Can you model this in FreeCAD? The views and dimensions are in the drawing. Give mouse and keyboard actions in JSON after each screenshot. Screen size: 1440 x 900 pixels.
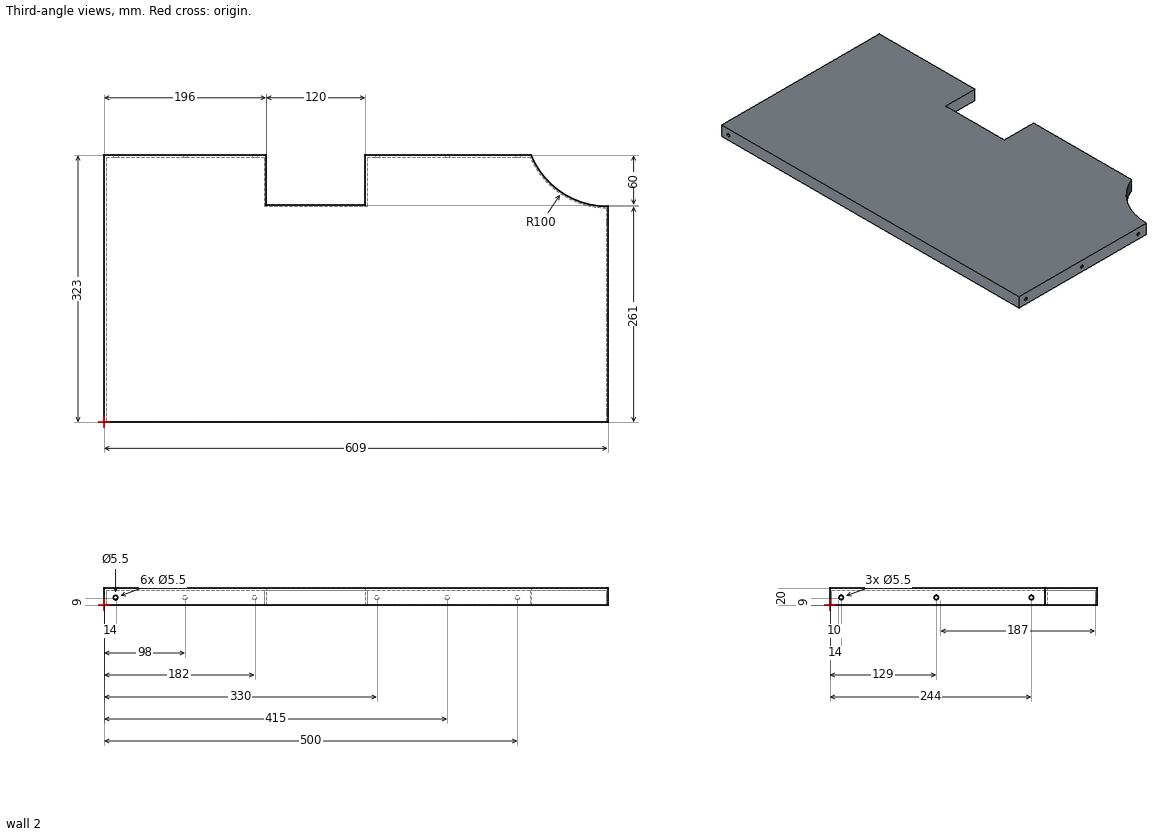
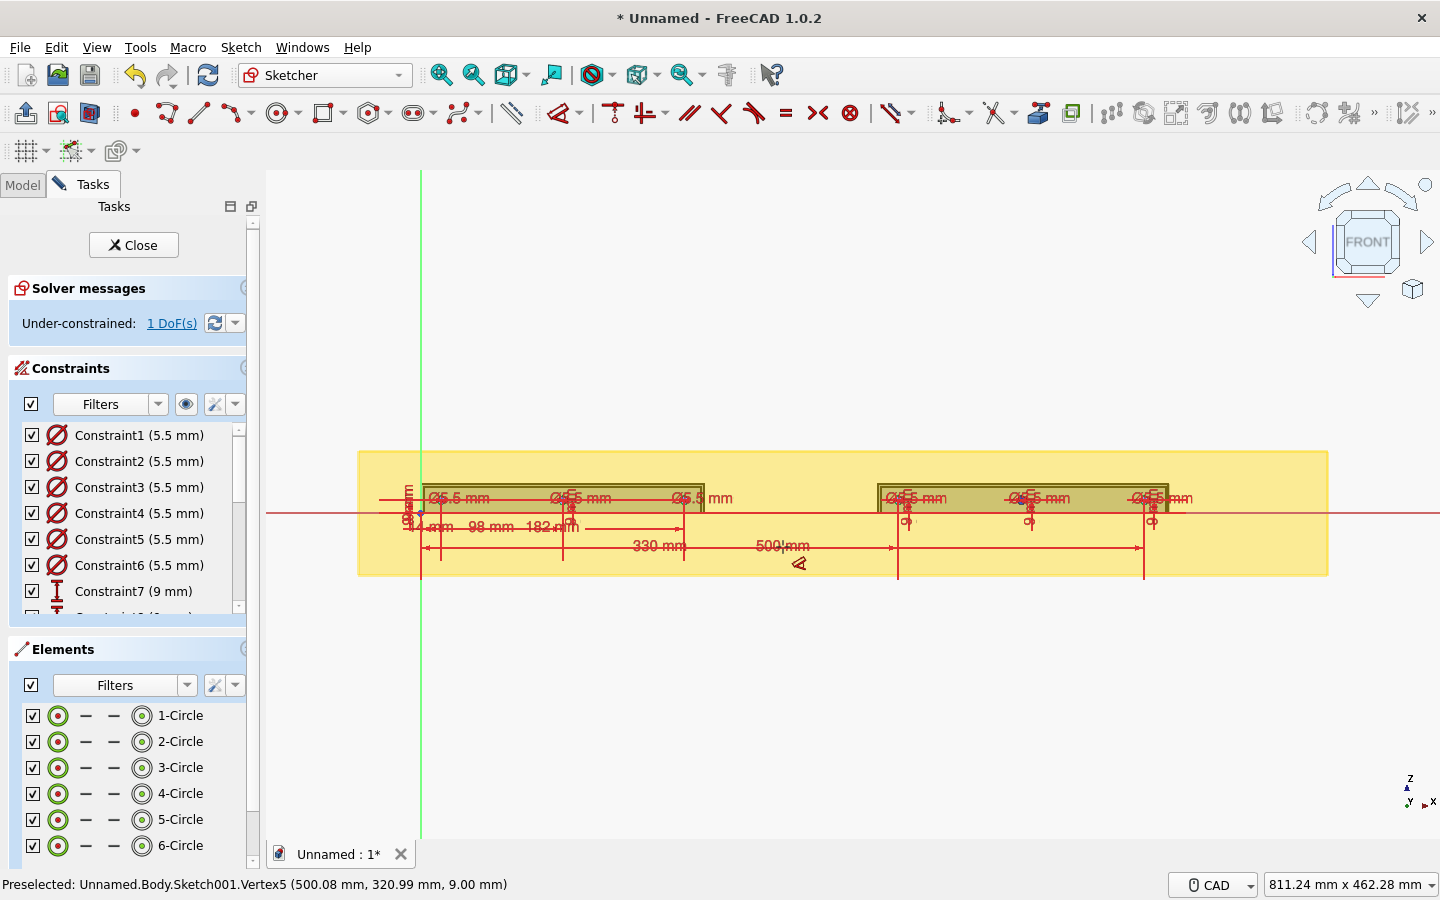
{"action": "left_click", "coordinate": [1021, 500]}
{"action": "left_click", "coordinate": [859, 547]}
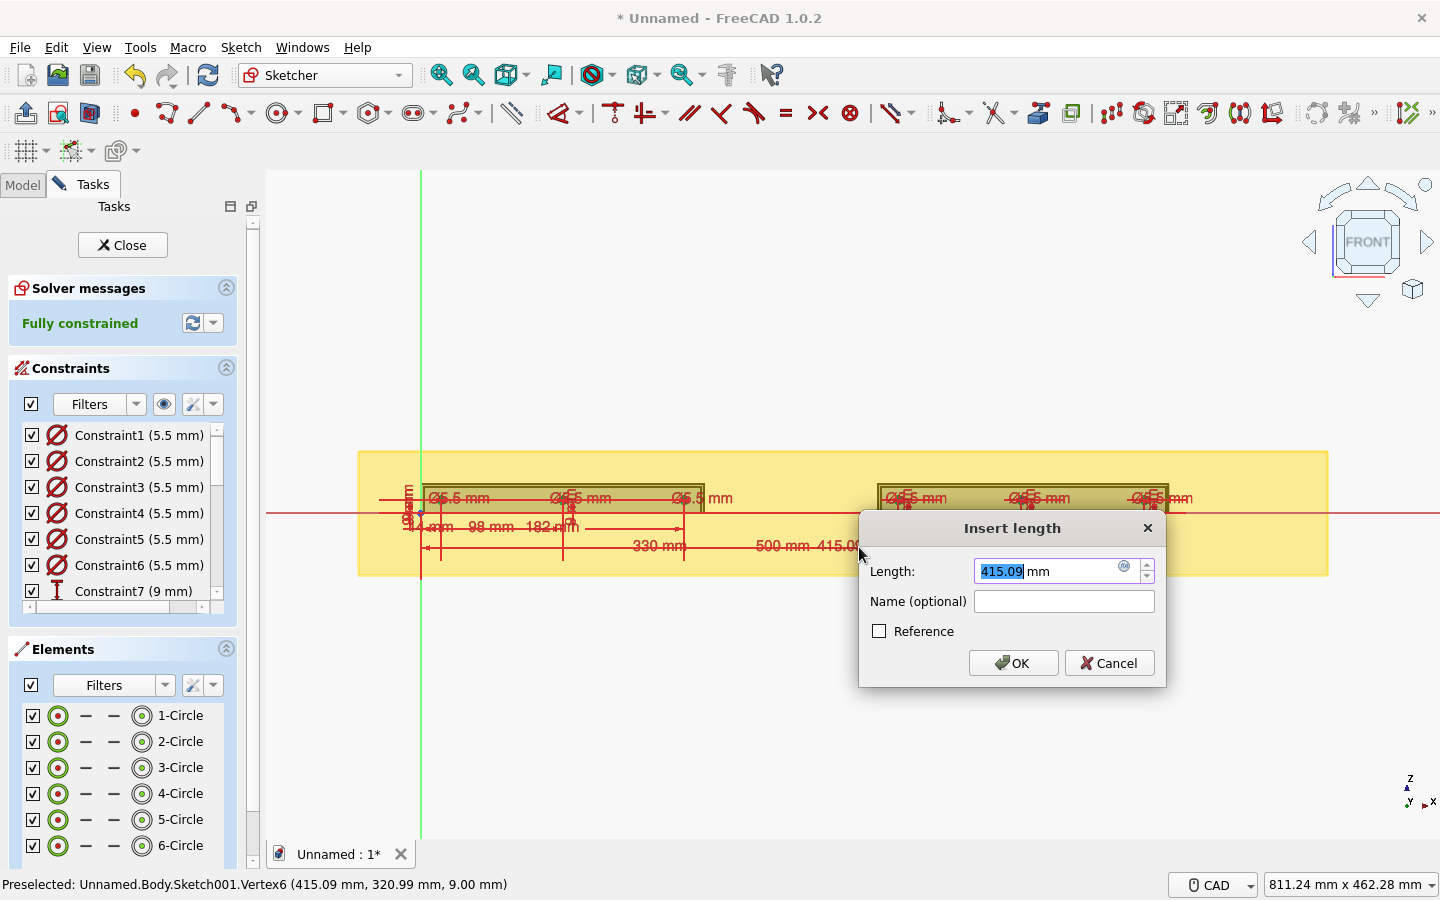
{"action": "type", "text": "415"}
{"action": "key", "text": "Return"}
{"action": "key", "text": "Escape"}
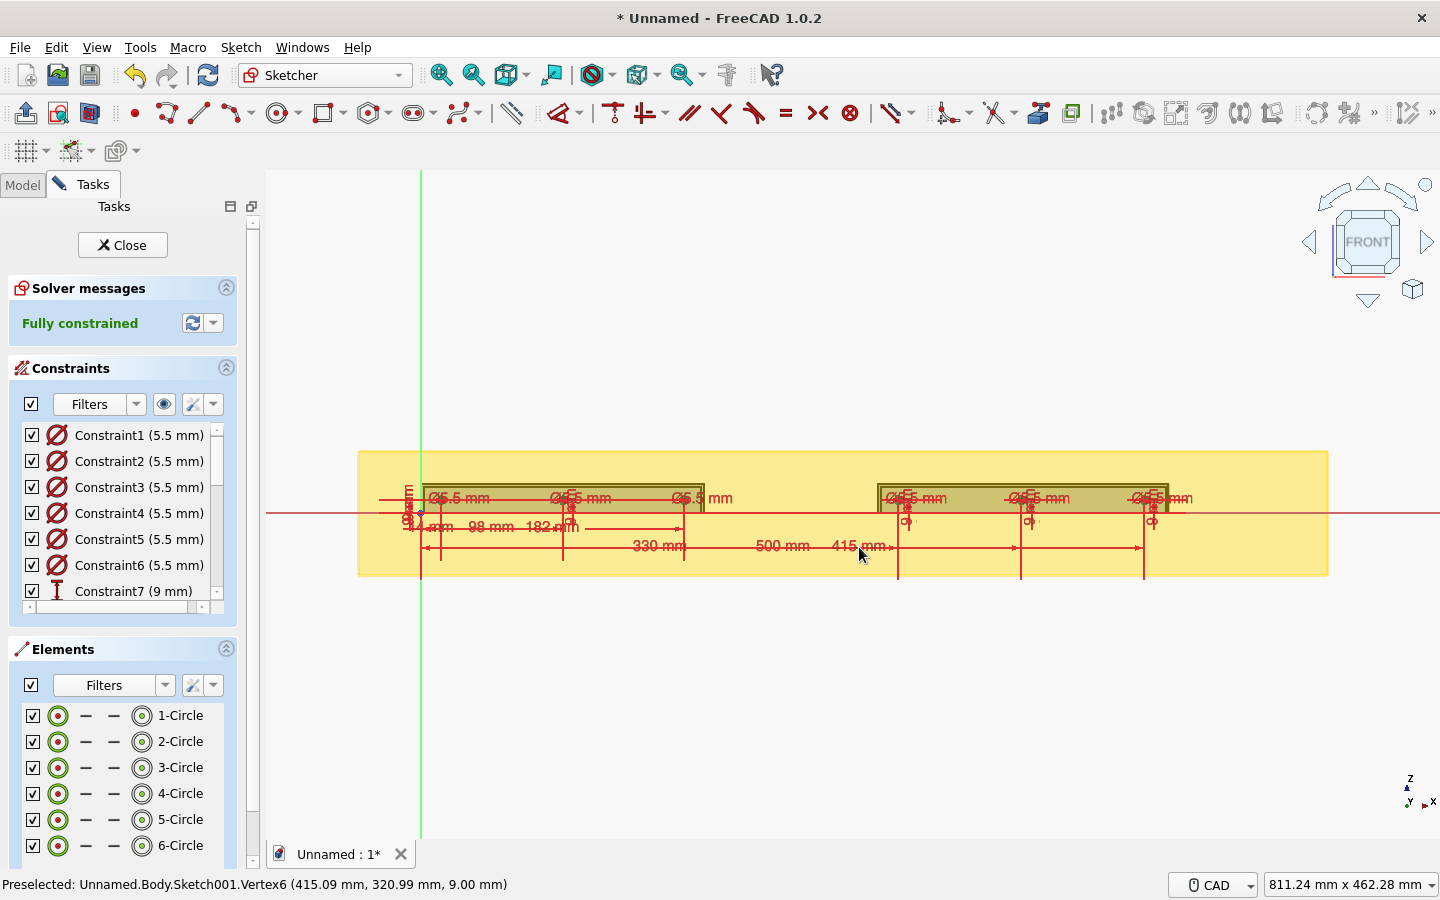
{"action": "left_click", "coordinate": [123, 245]}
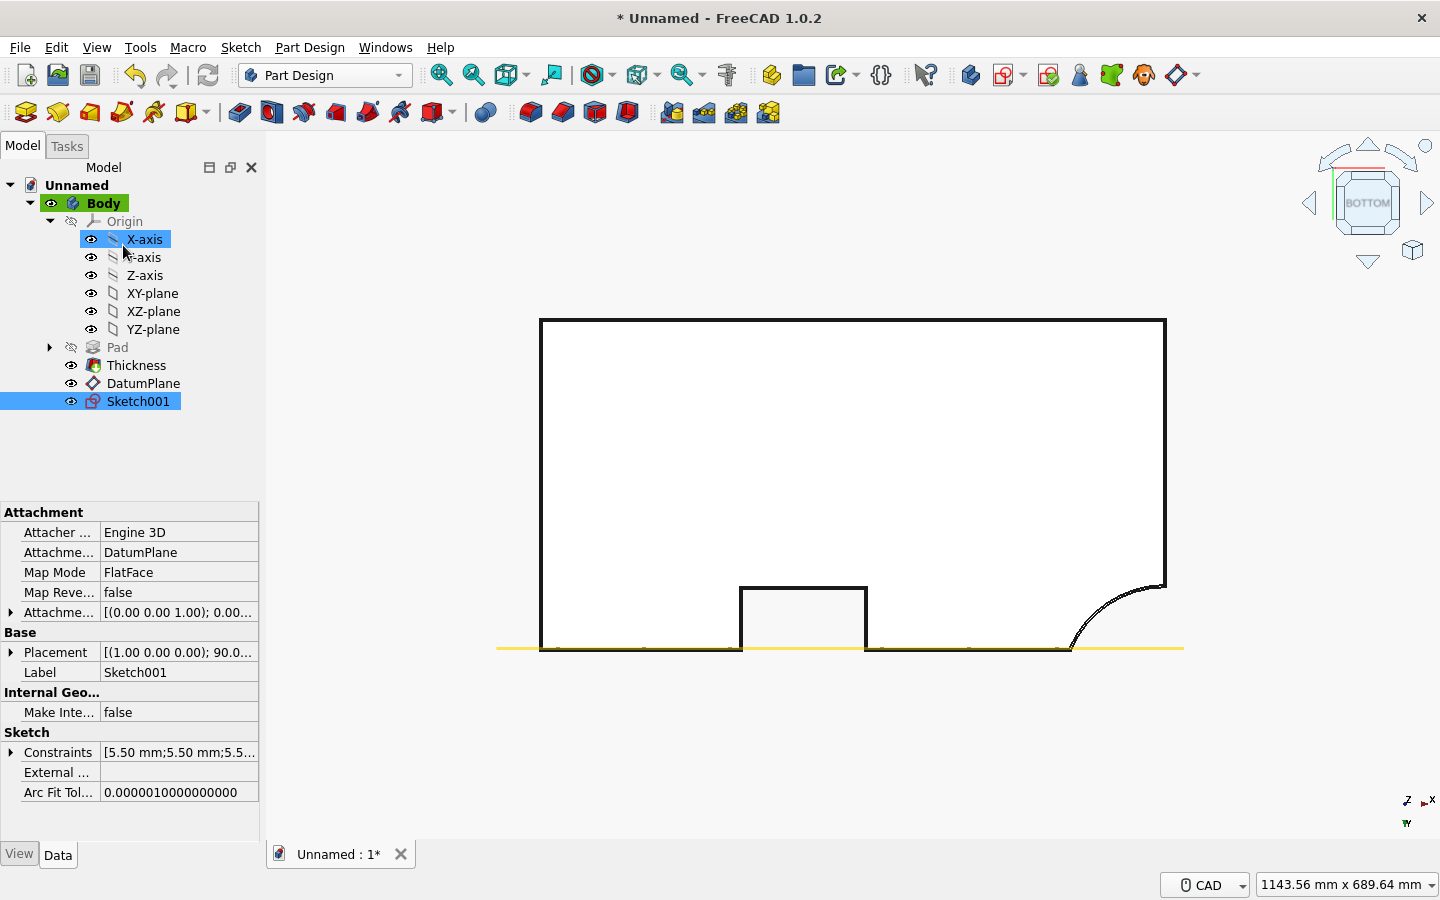
{"action": "left_click", "coordinate": [240, 112]}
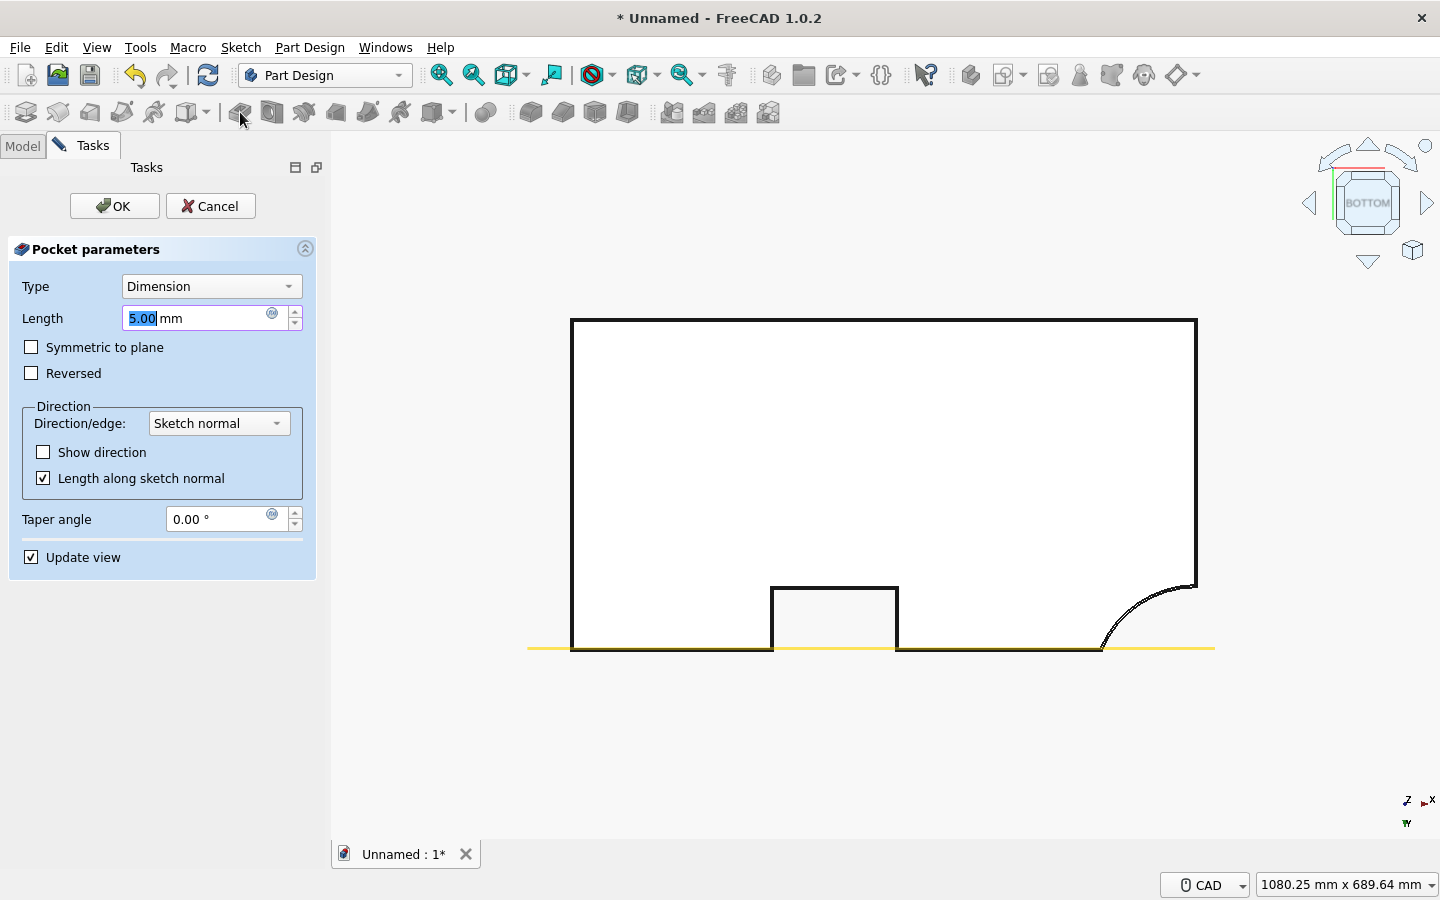
{"action": "left_click", "coordinate": [212, 286]}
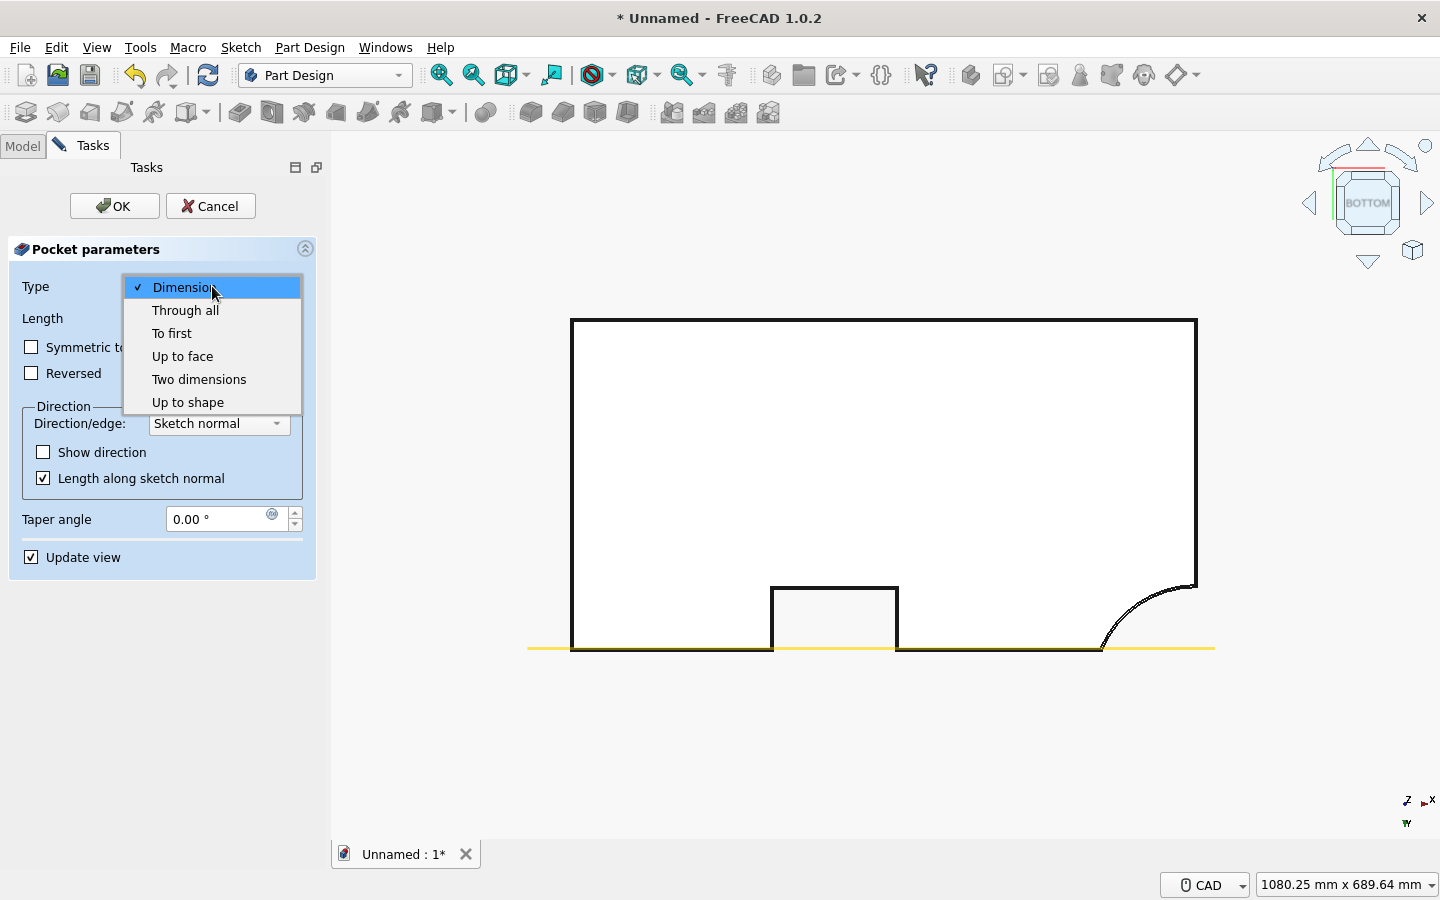
{"action": "left_click", "coordinate": [212, 380]}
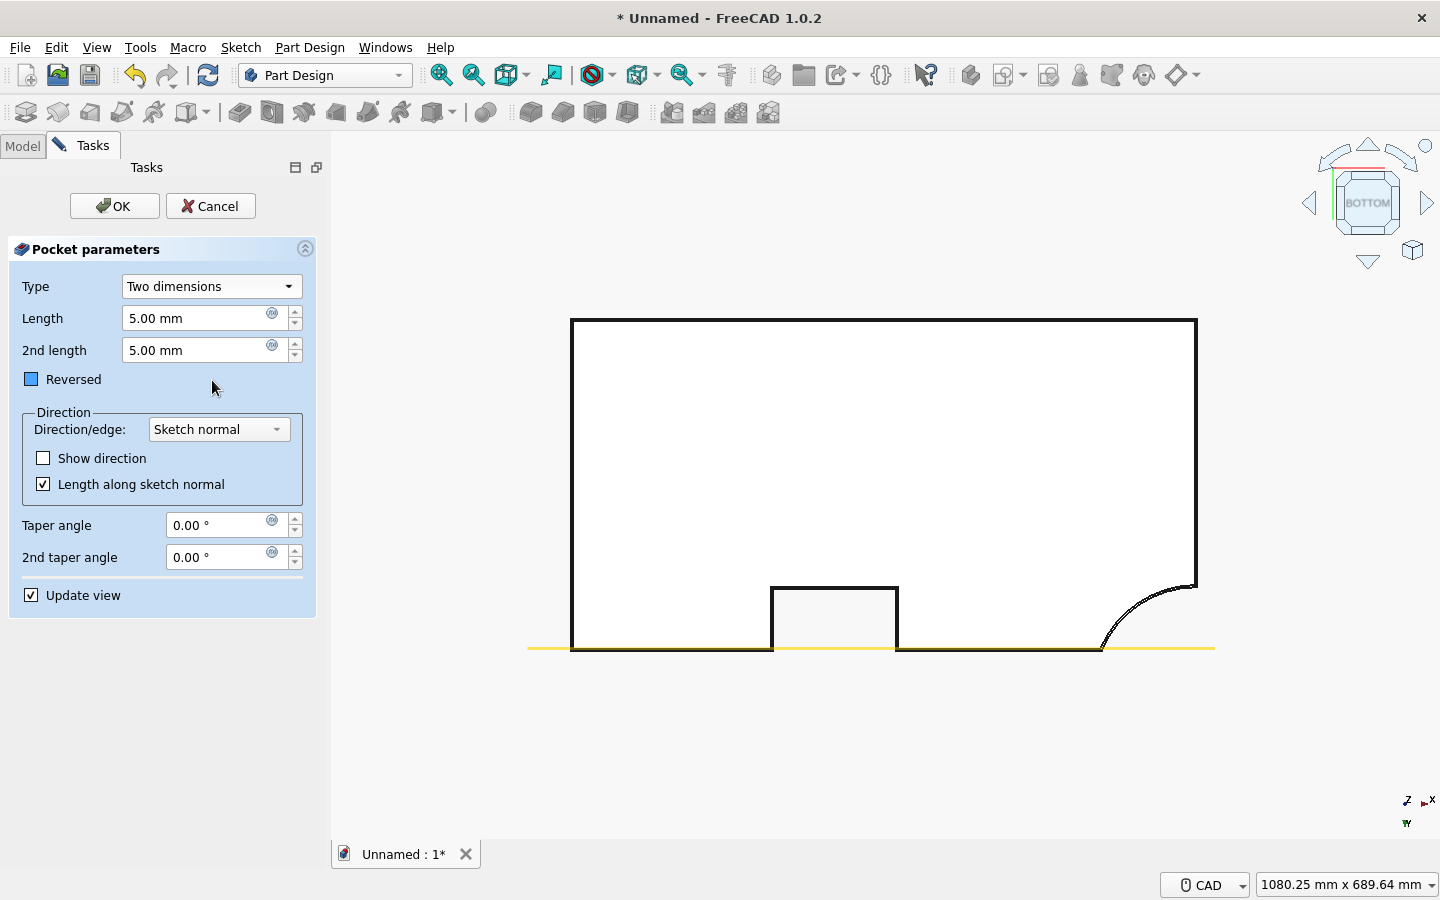
{"action": "triple_click", "coordinate": [204, 318]}